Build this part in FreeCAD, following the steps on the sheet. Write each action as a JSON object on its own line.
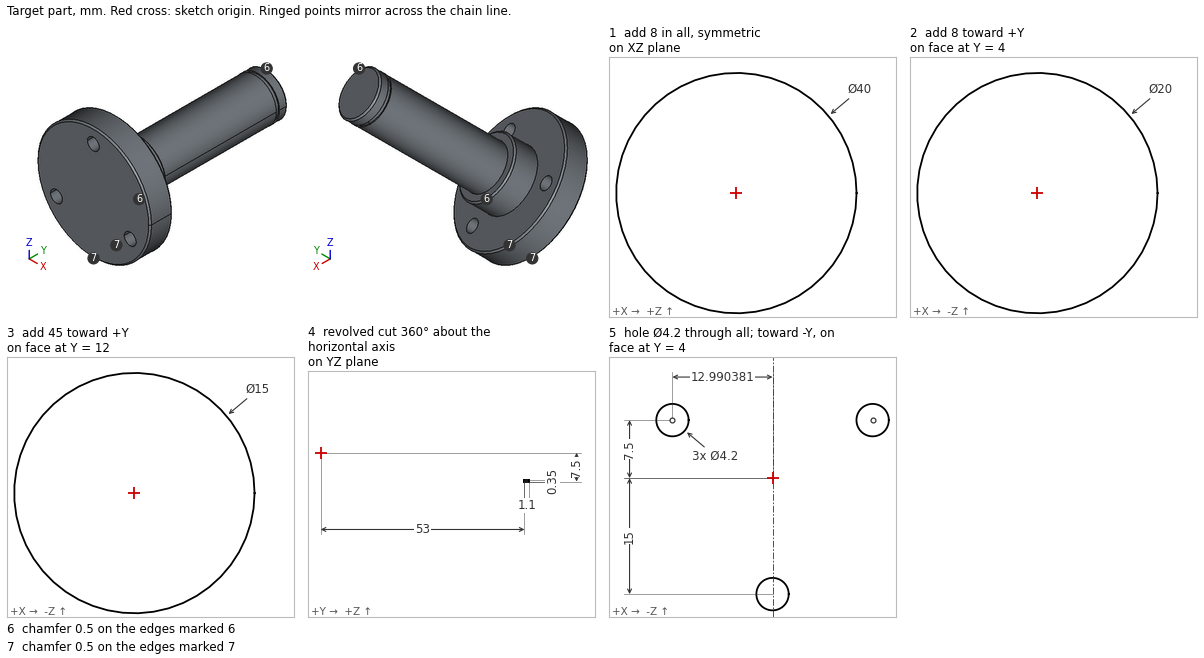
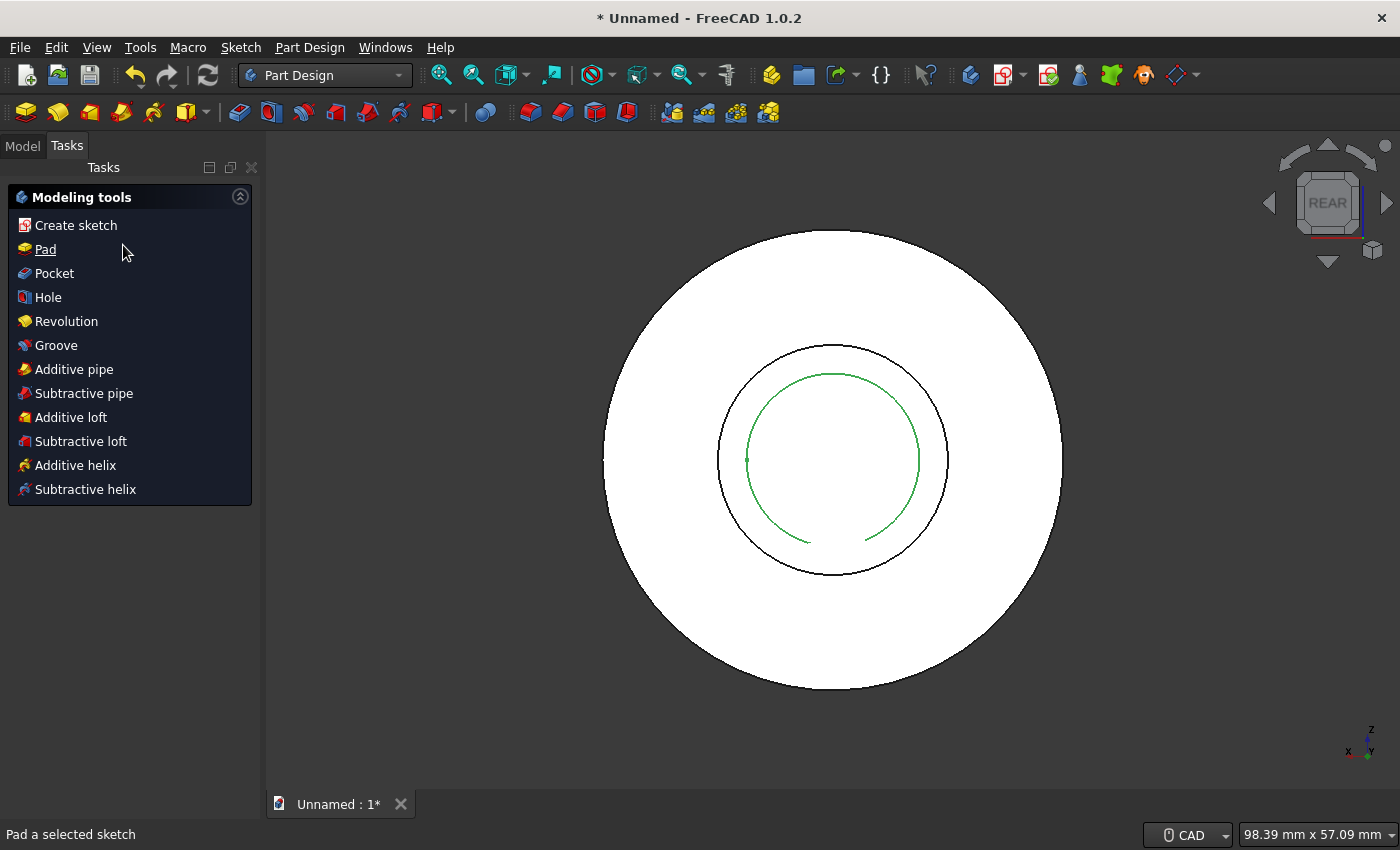
{"action": "left_click", "coordinate": [26, 112]}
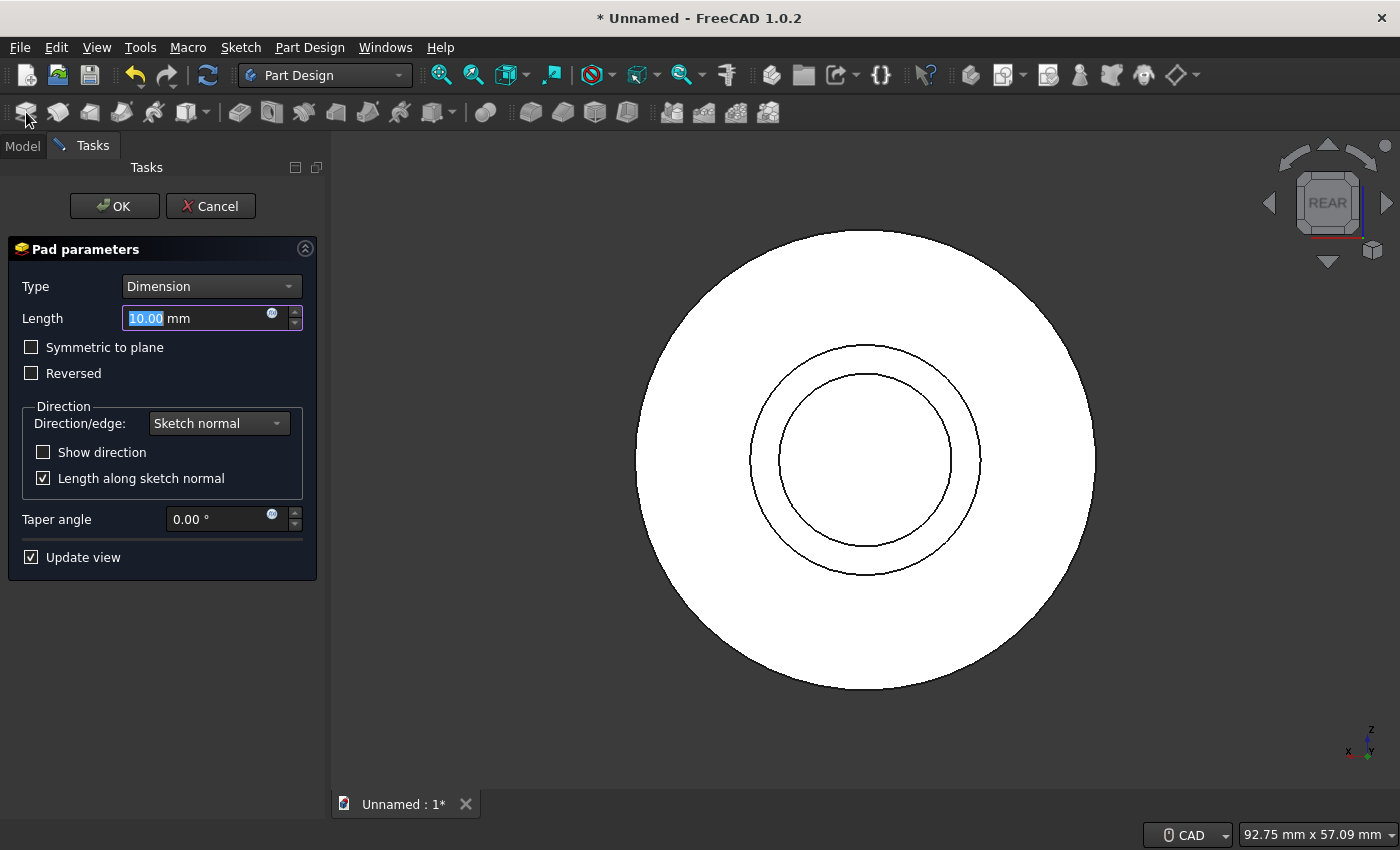
{"action": "type", "text": "45"}
{"action": "key", "text": "Tab"}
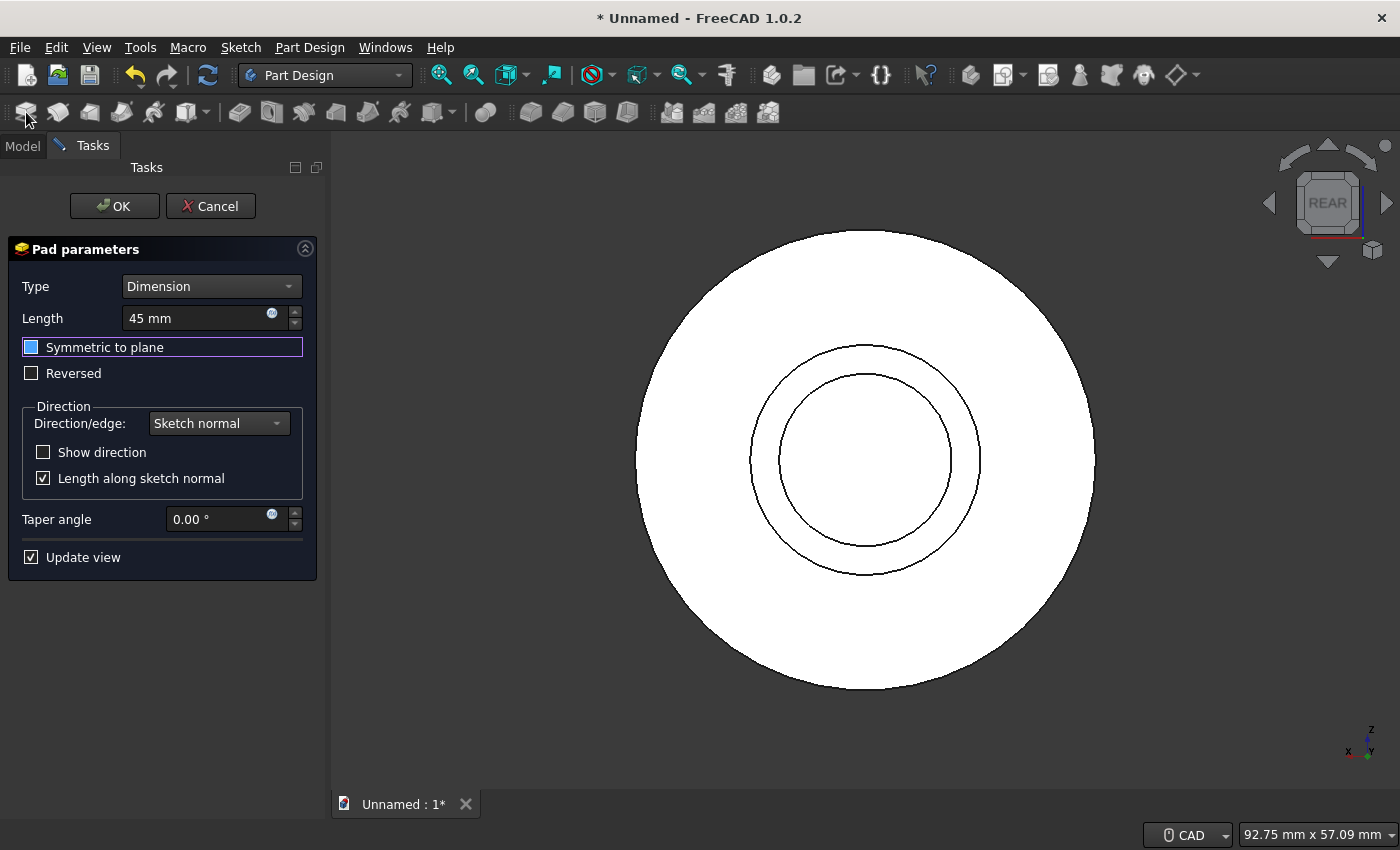
{"action": "left_click", "coordinate": [115, 206]}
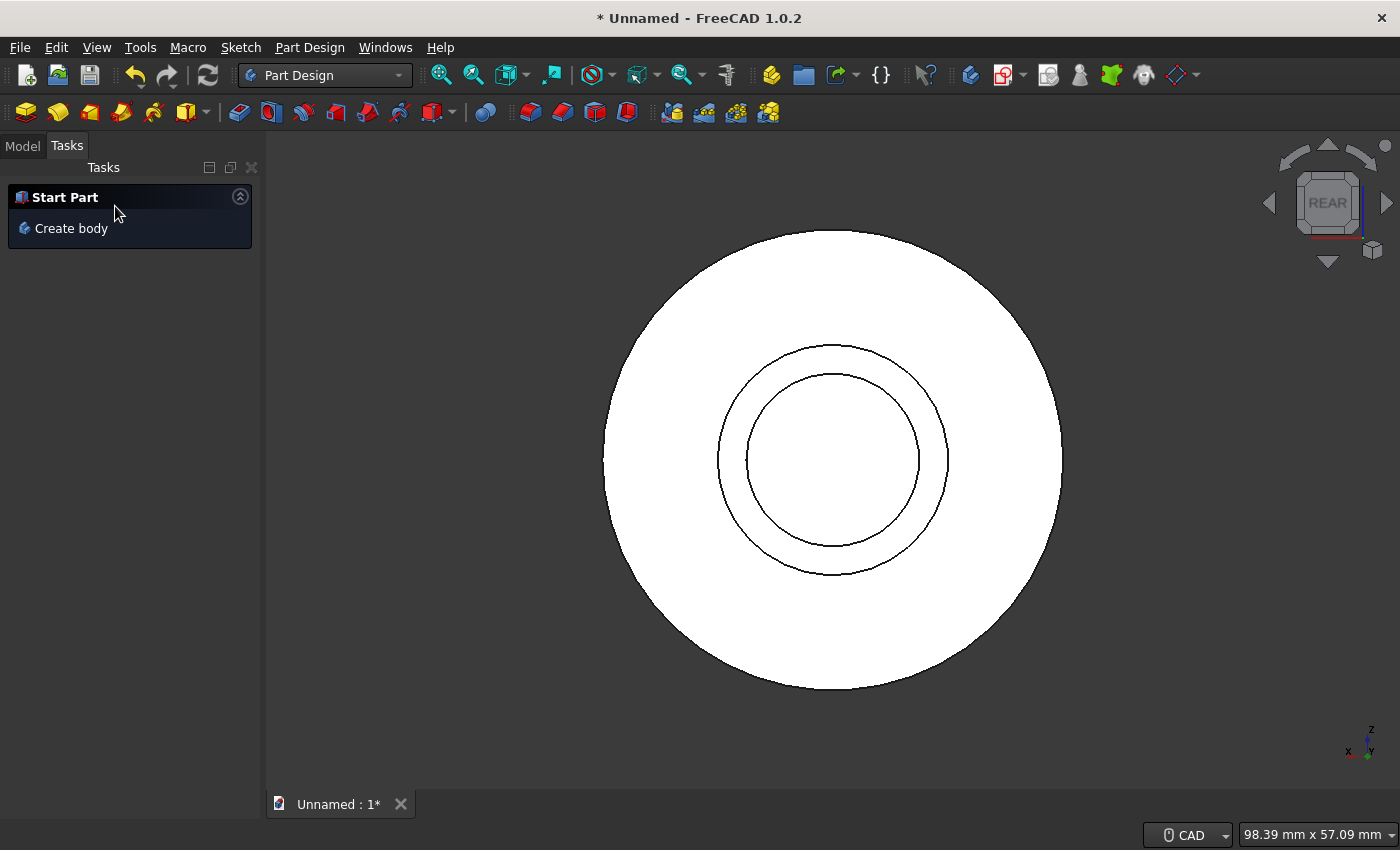
{"action": "left_click", "coordinate": [1004, 76]}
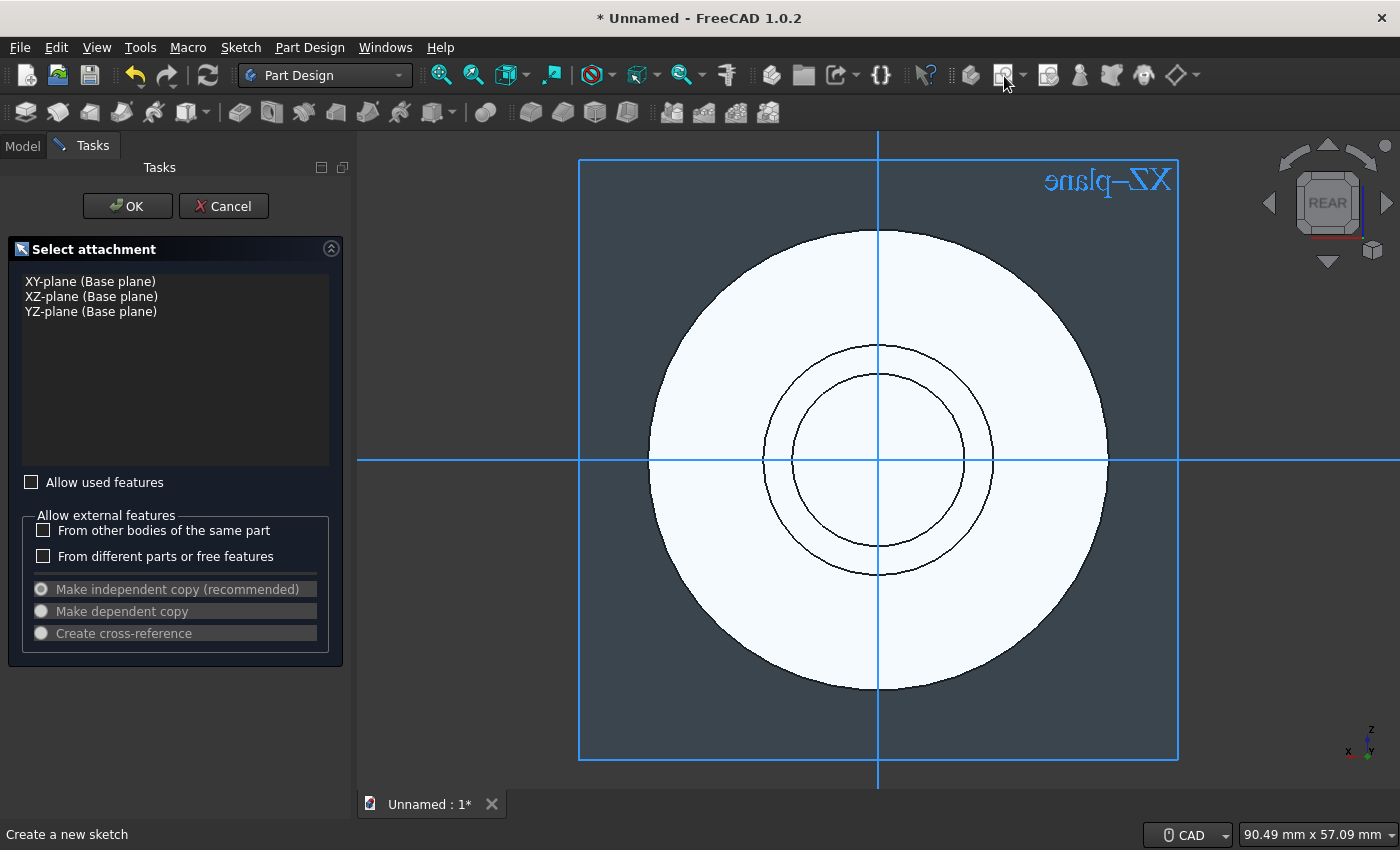
{"action": "left_click", "coordinate": [82, 312]}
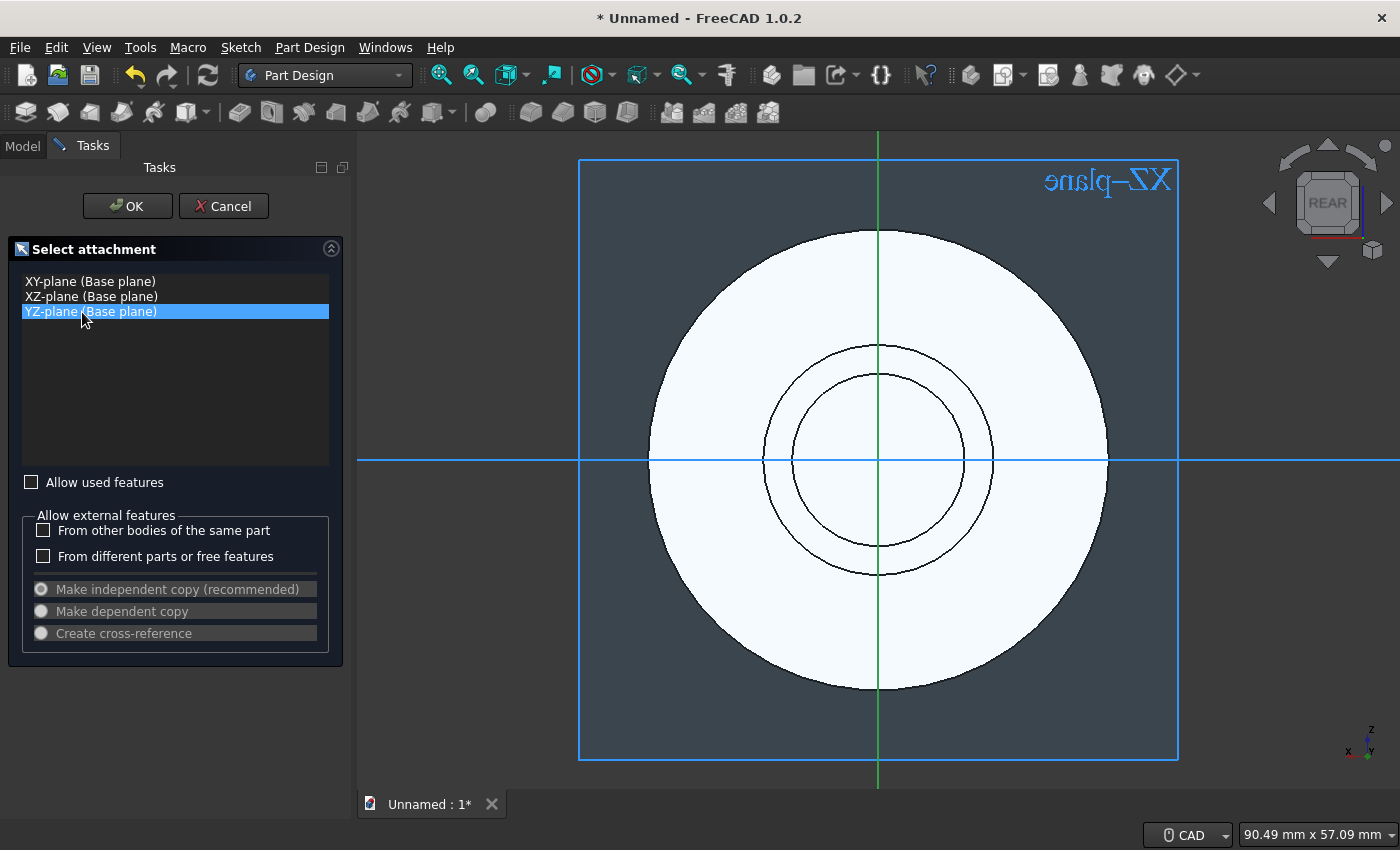
{"action": "left_click", "coordinate": [128, 206]}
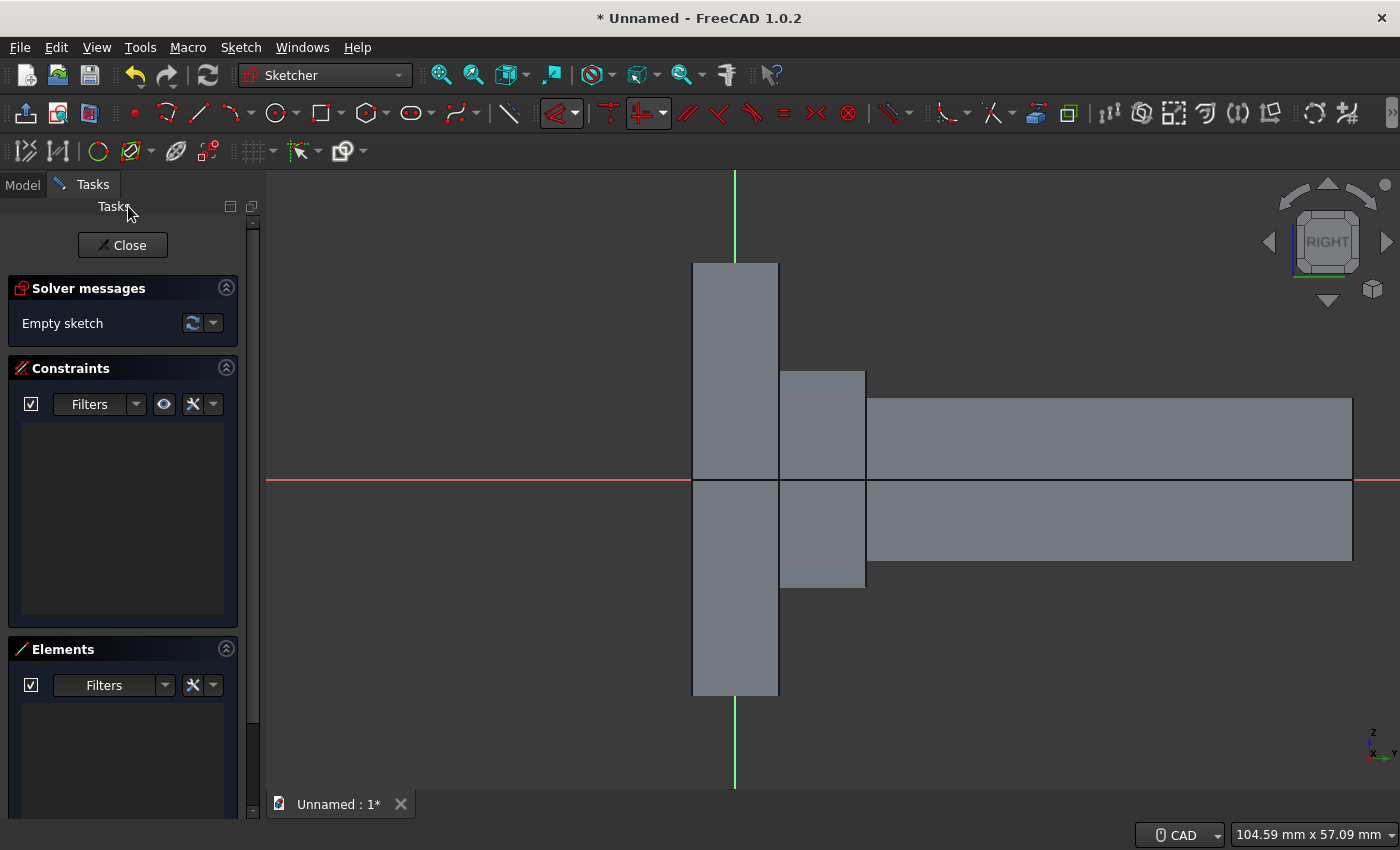
{"action": "left_click", "coordinate": [90, 114]}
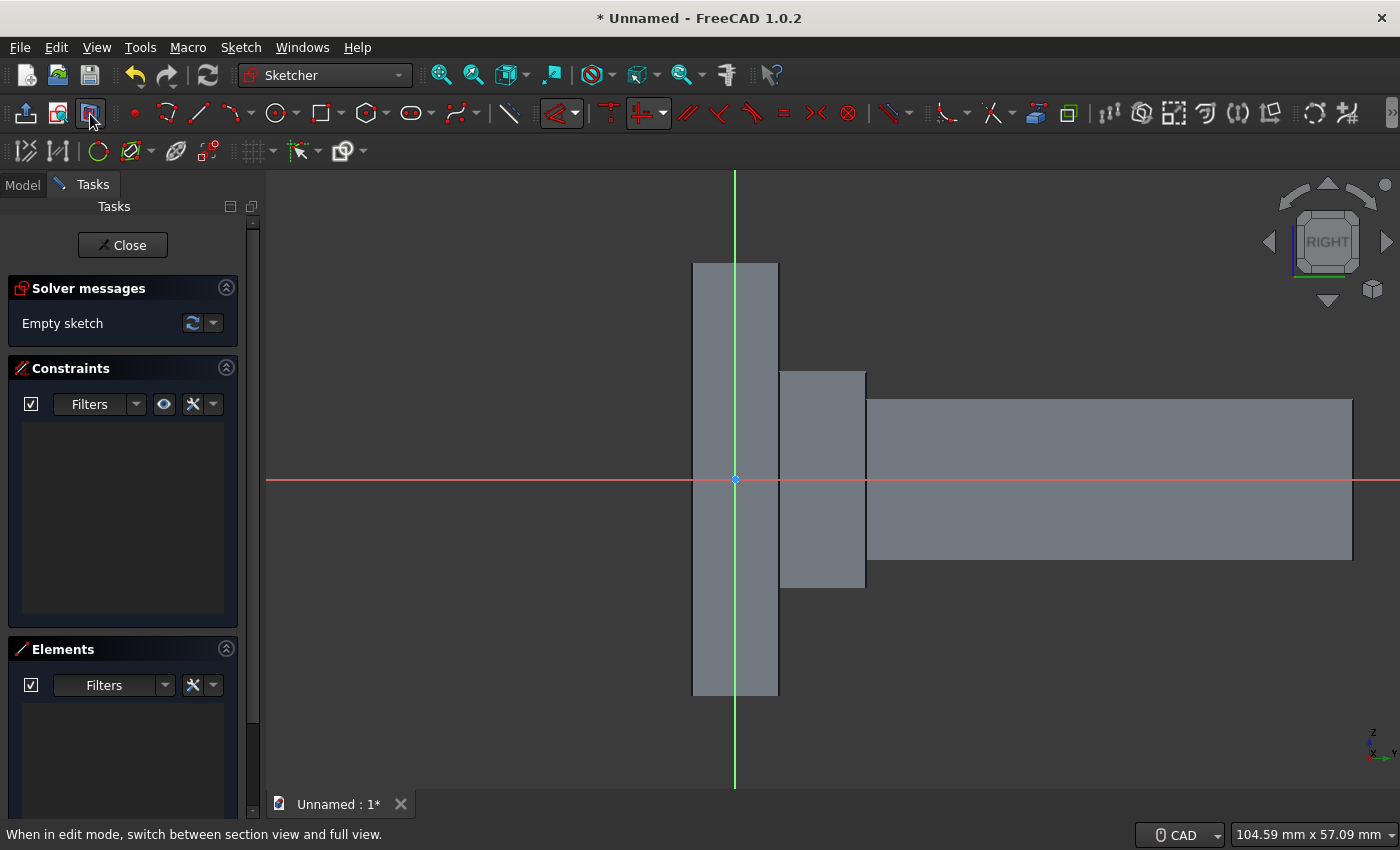
{"action": "scroll", "coordinate": [764, 480], "scroll_direction": "down", "scroll_amount": 5}